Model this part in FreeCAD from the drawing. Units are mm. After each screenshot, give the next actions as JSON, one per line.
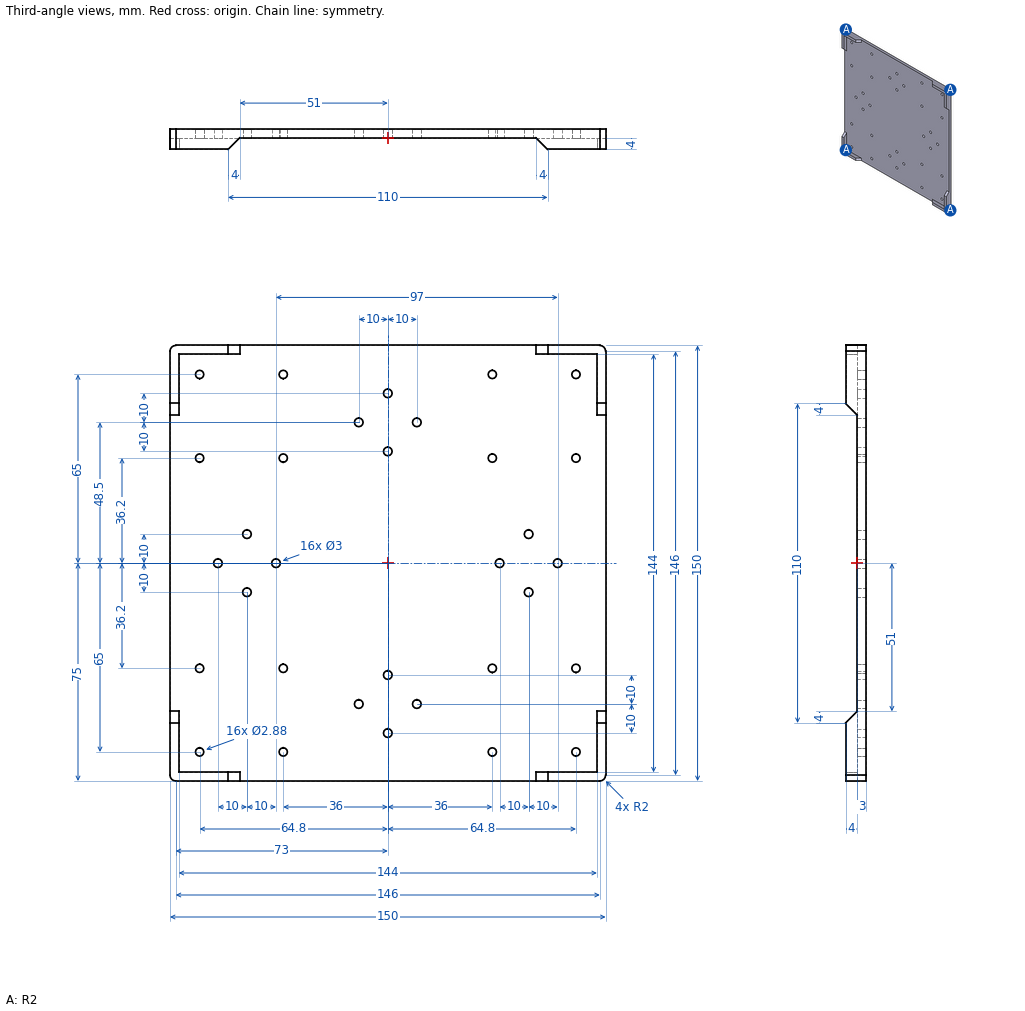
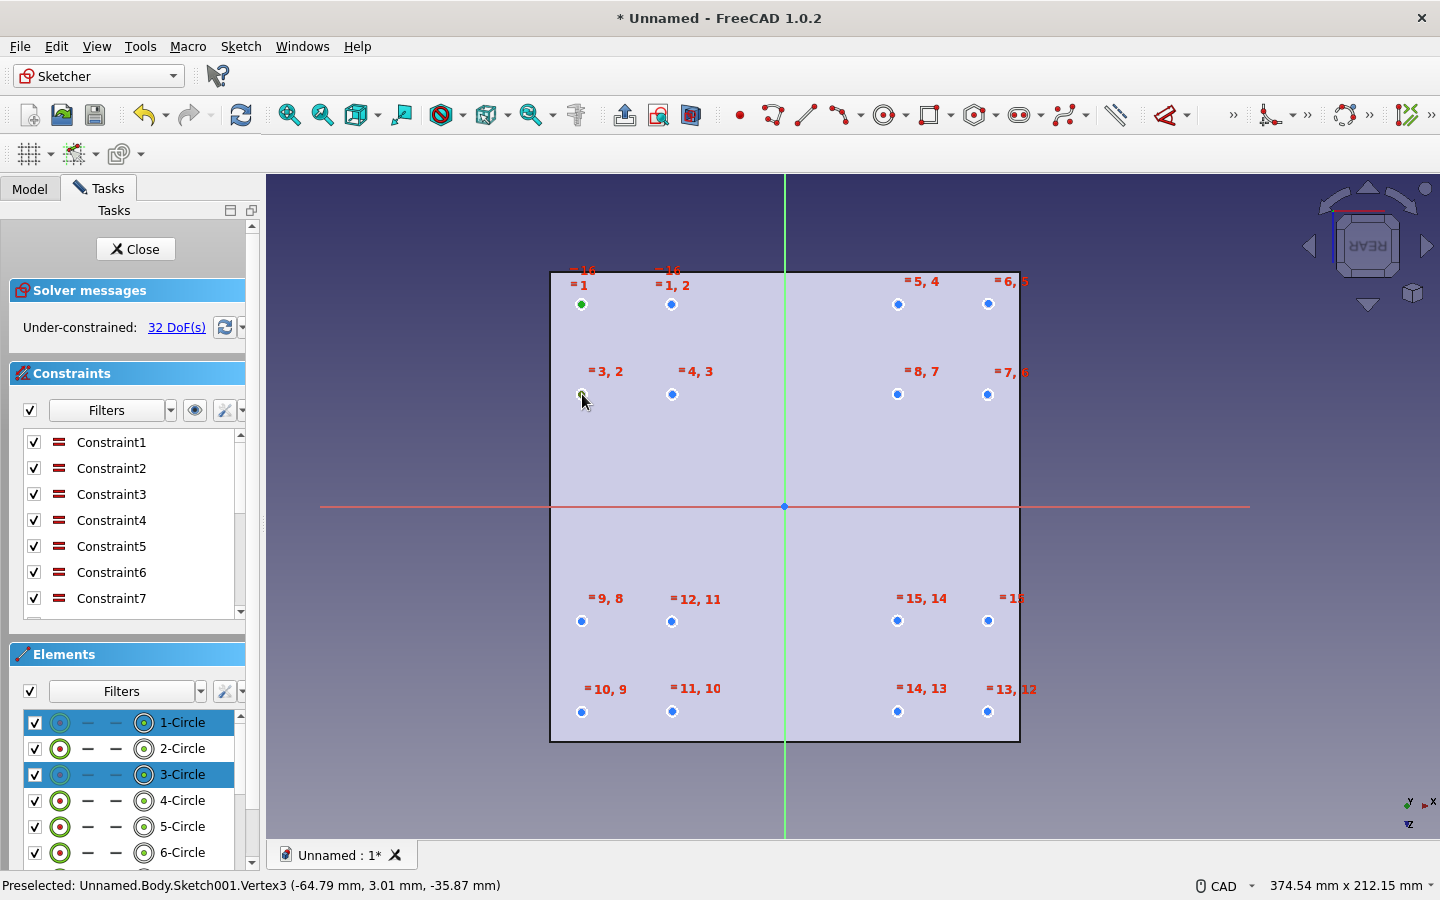
{"action": "key", "text": "v"}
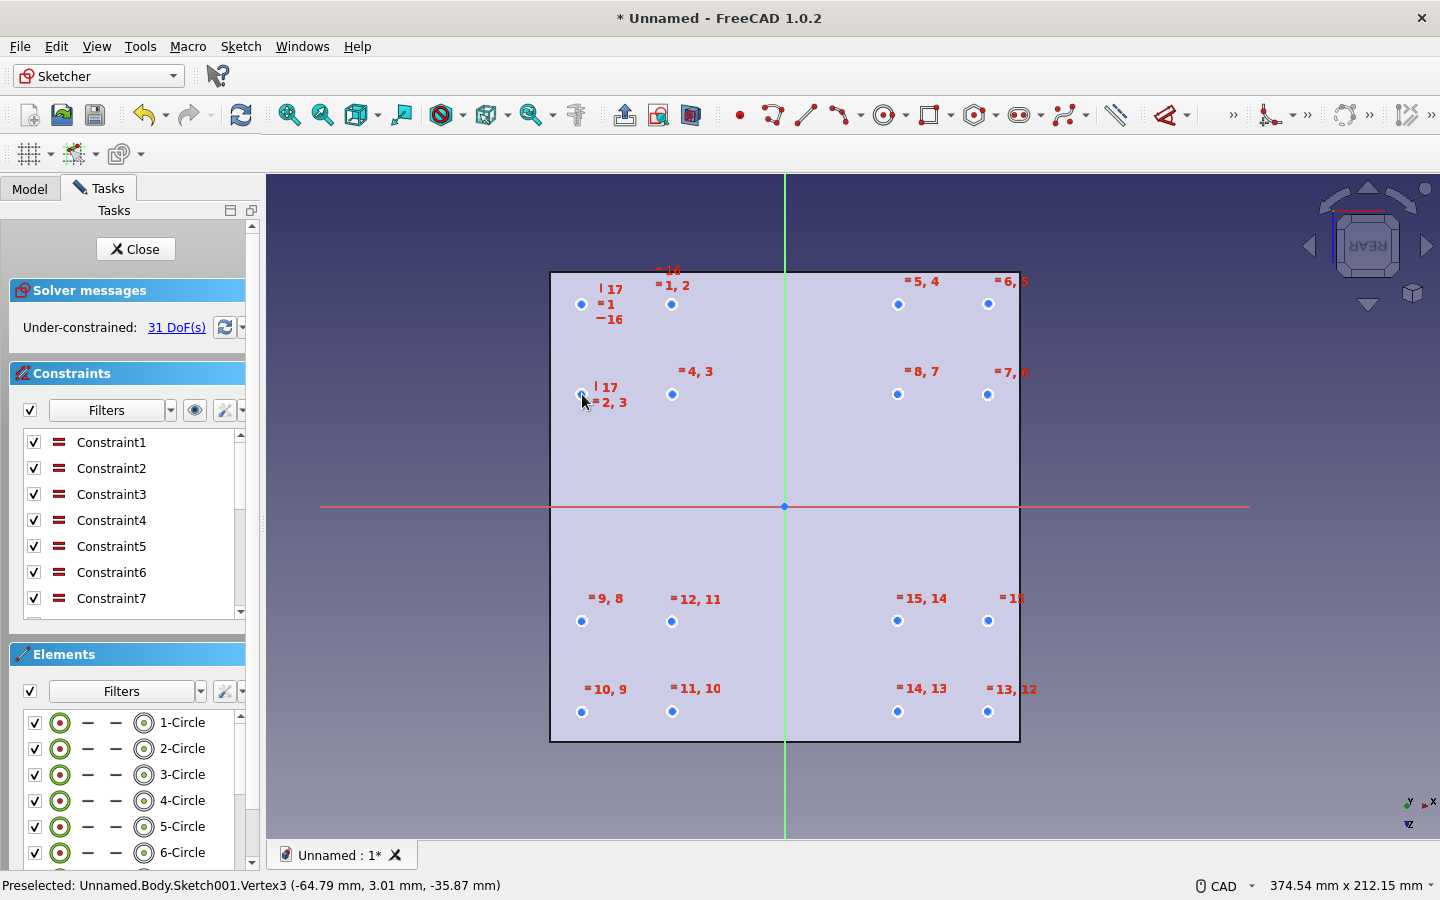
{"action": "left_click", "coordinate": [672, 304]}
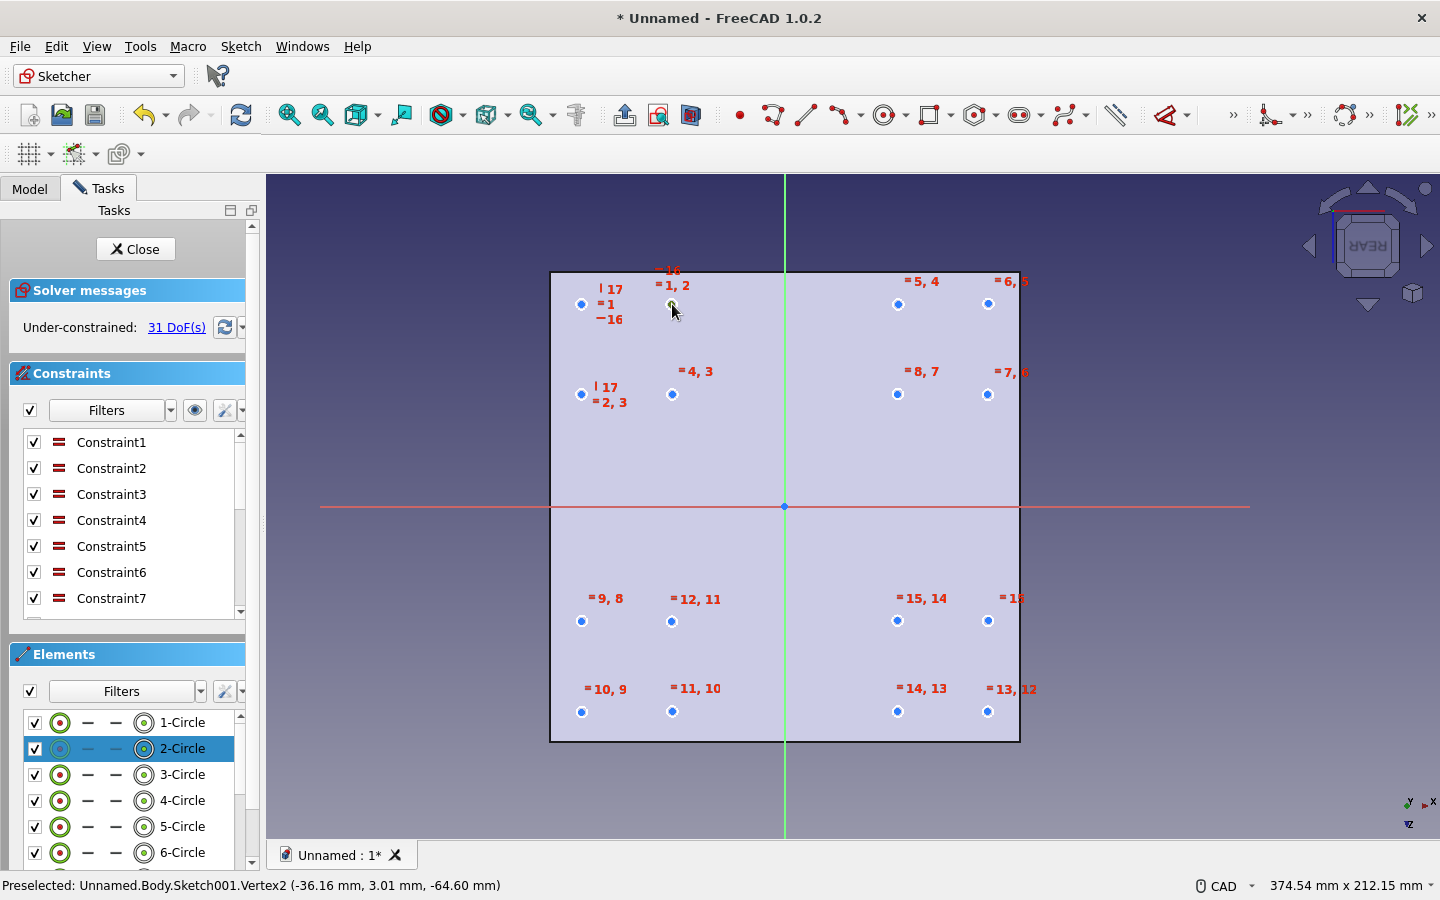
{"action": "left_click", "coordinate": [672, 394]}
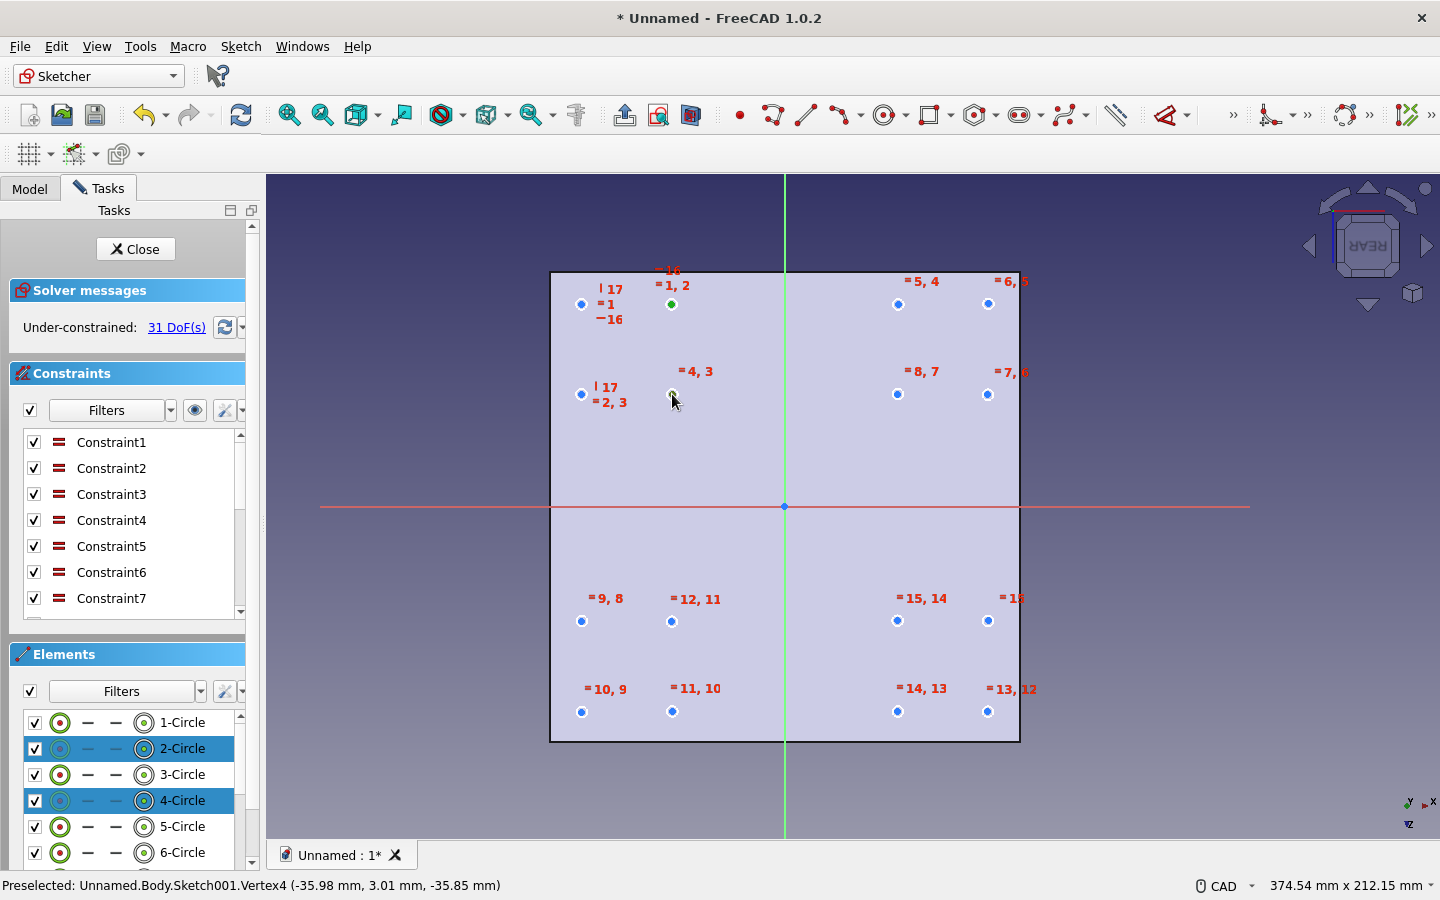
{"action": "key", "text": "v"}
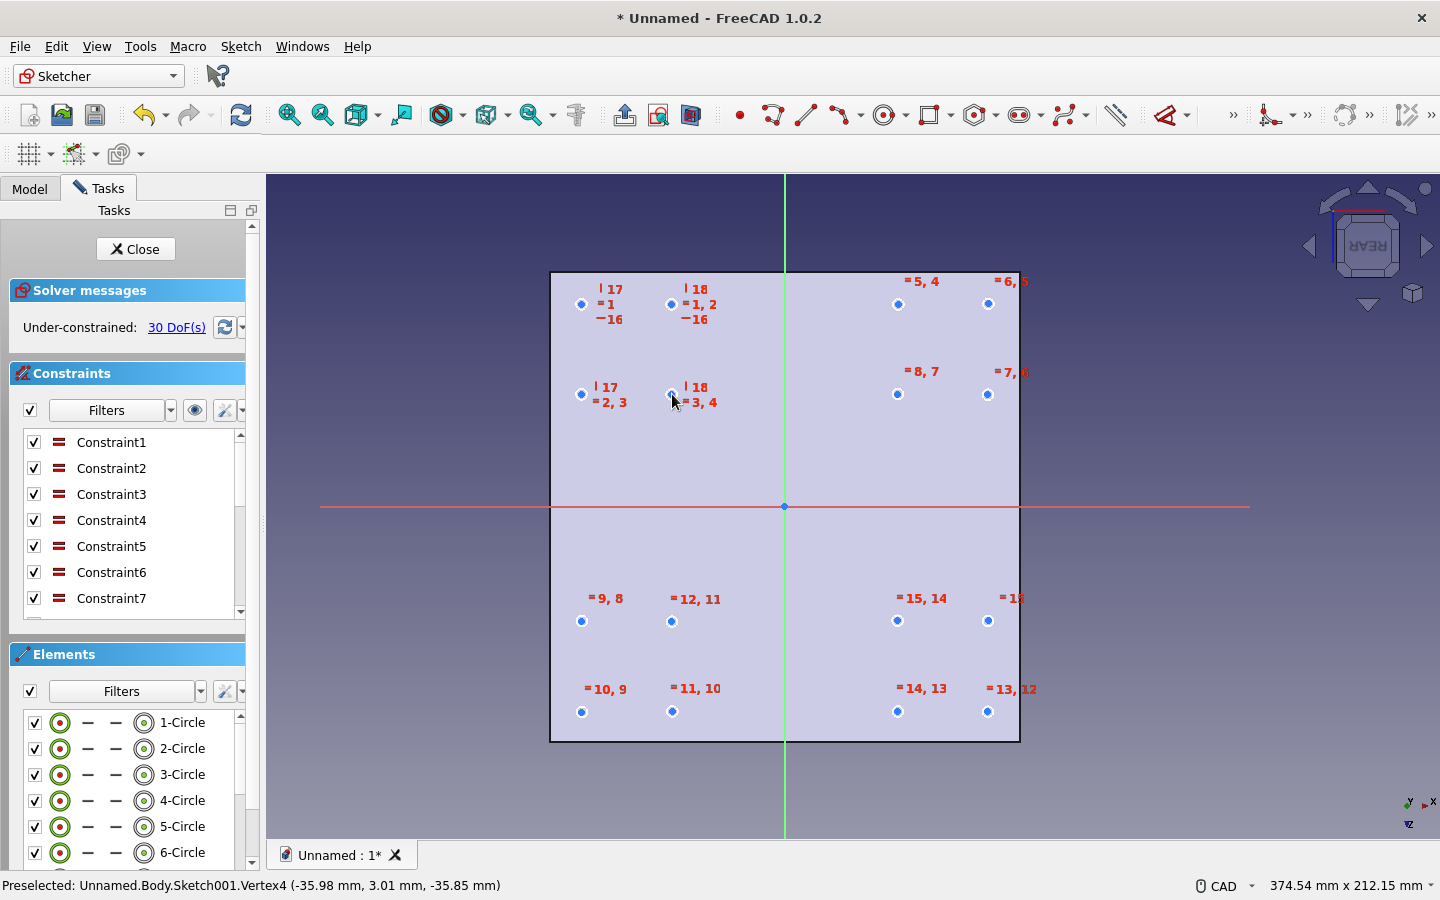
{"action": "left_click", "coordinate": [581, 394]}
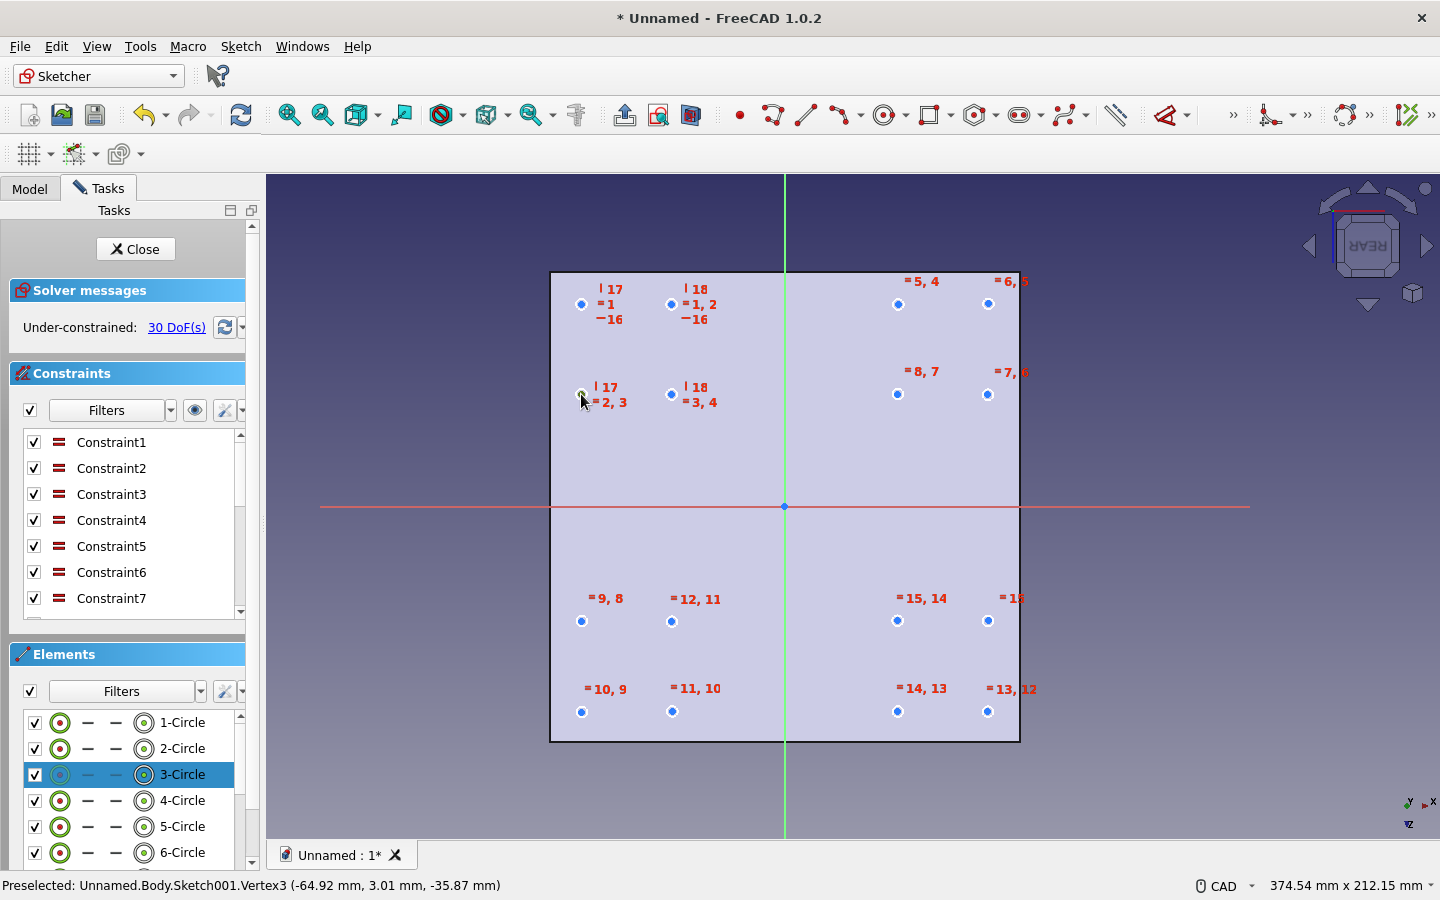
{"action": "left_click", "coordinate": [672, 394]}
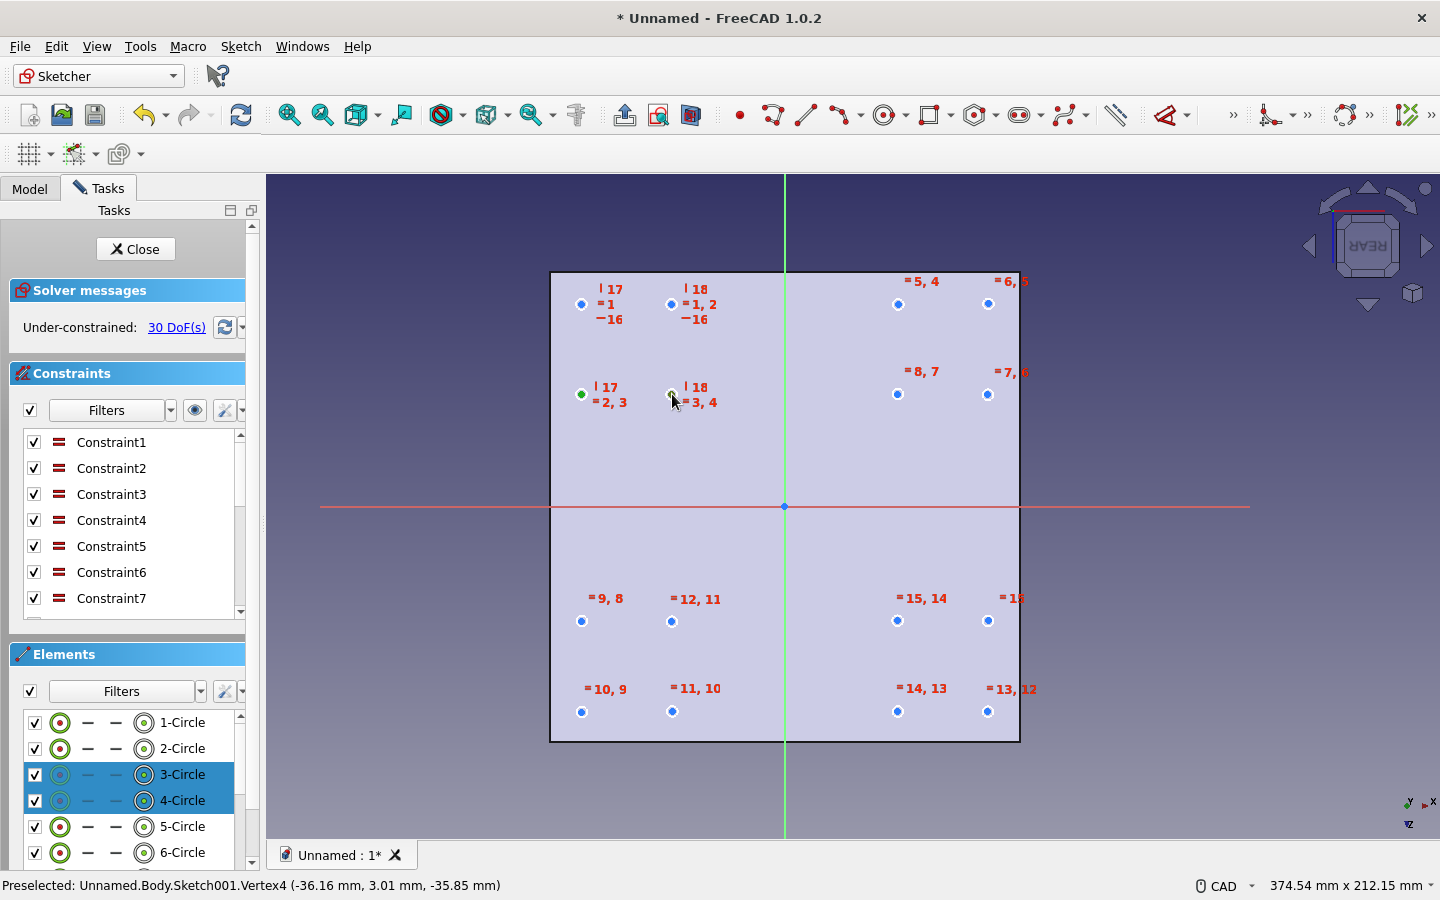
{"action": "key", "text": "h"}